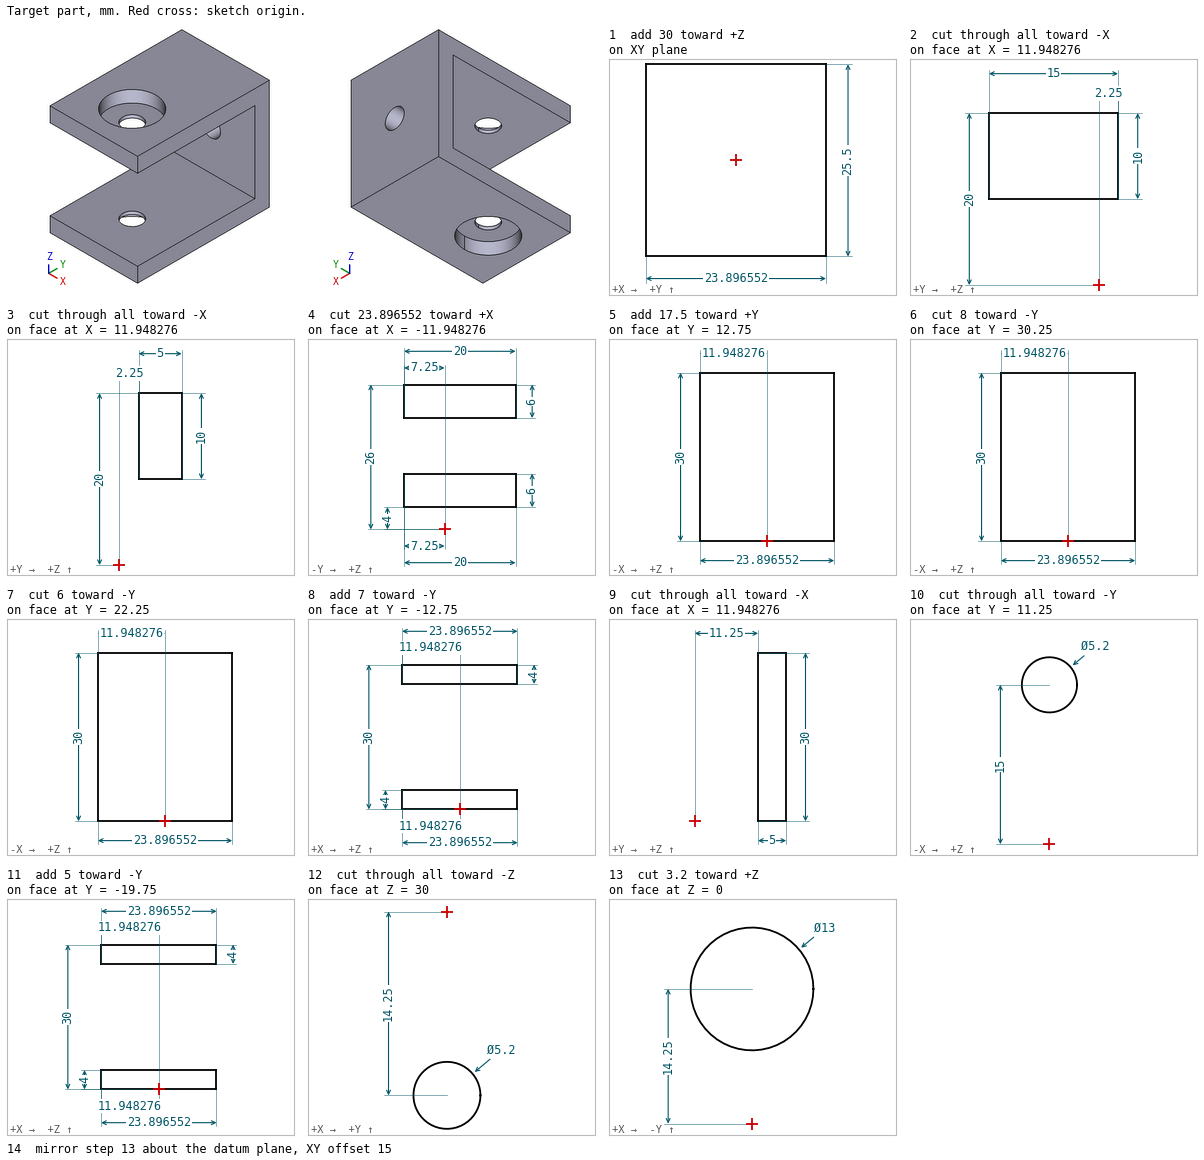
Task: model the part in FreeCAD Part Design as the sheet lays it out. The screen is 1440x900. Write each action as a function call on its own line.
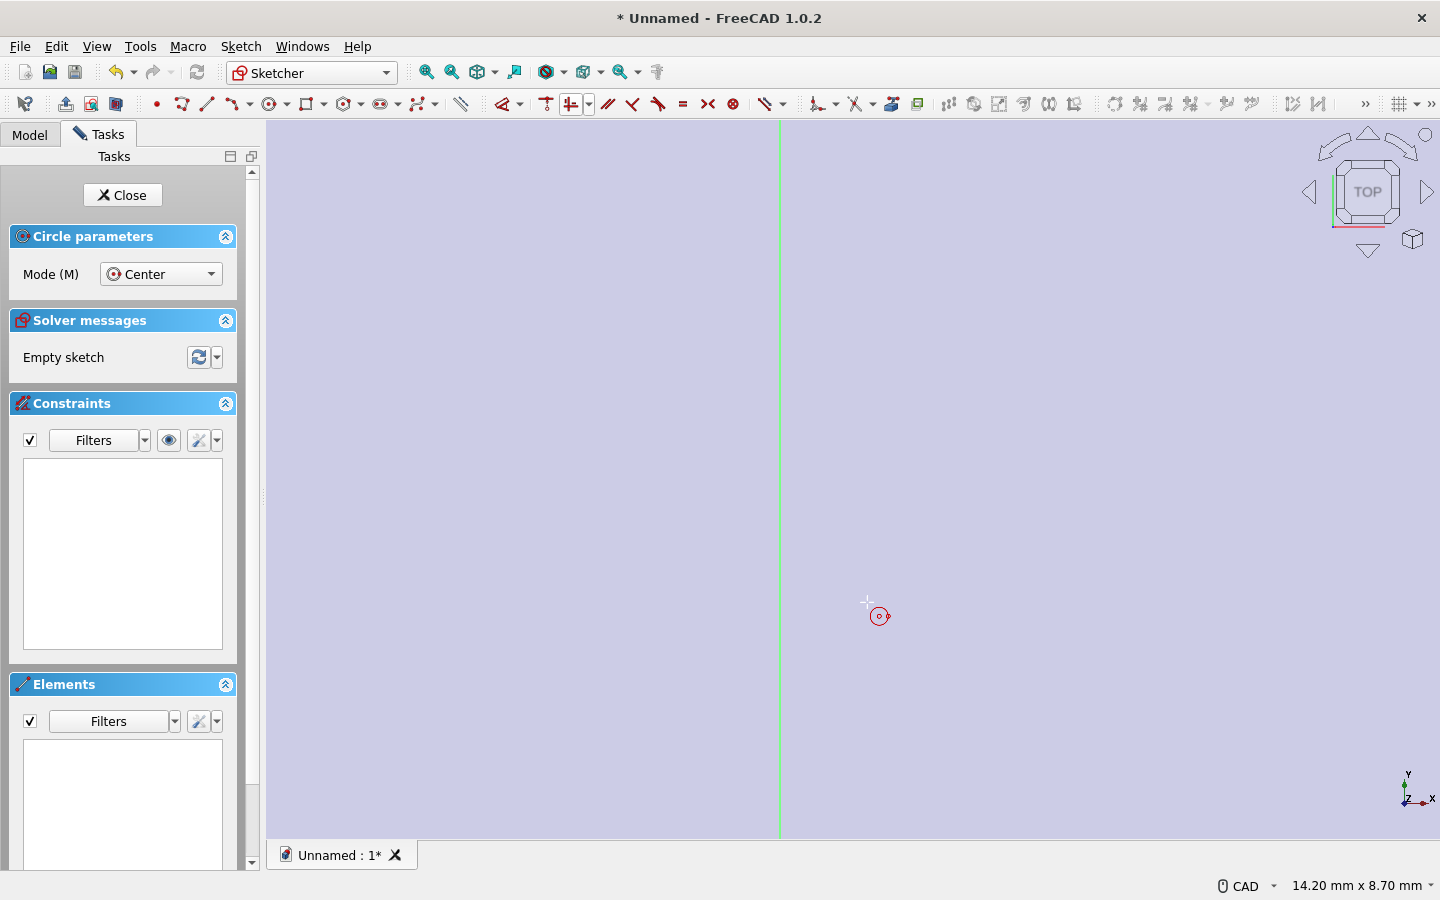
click(780, 478)
move(932, 326)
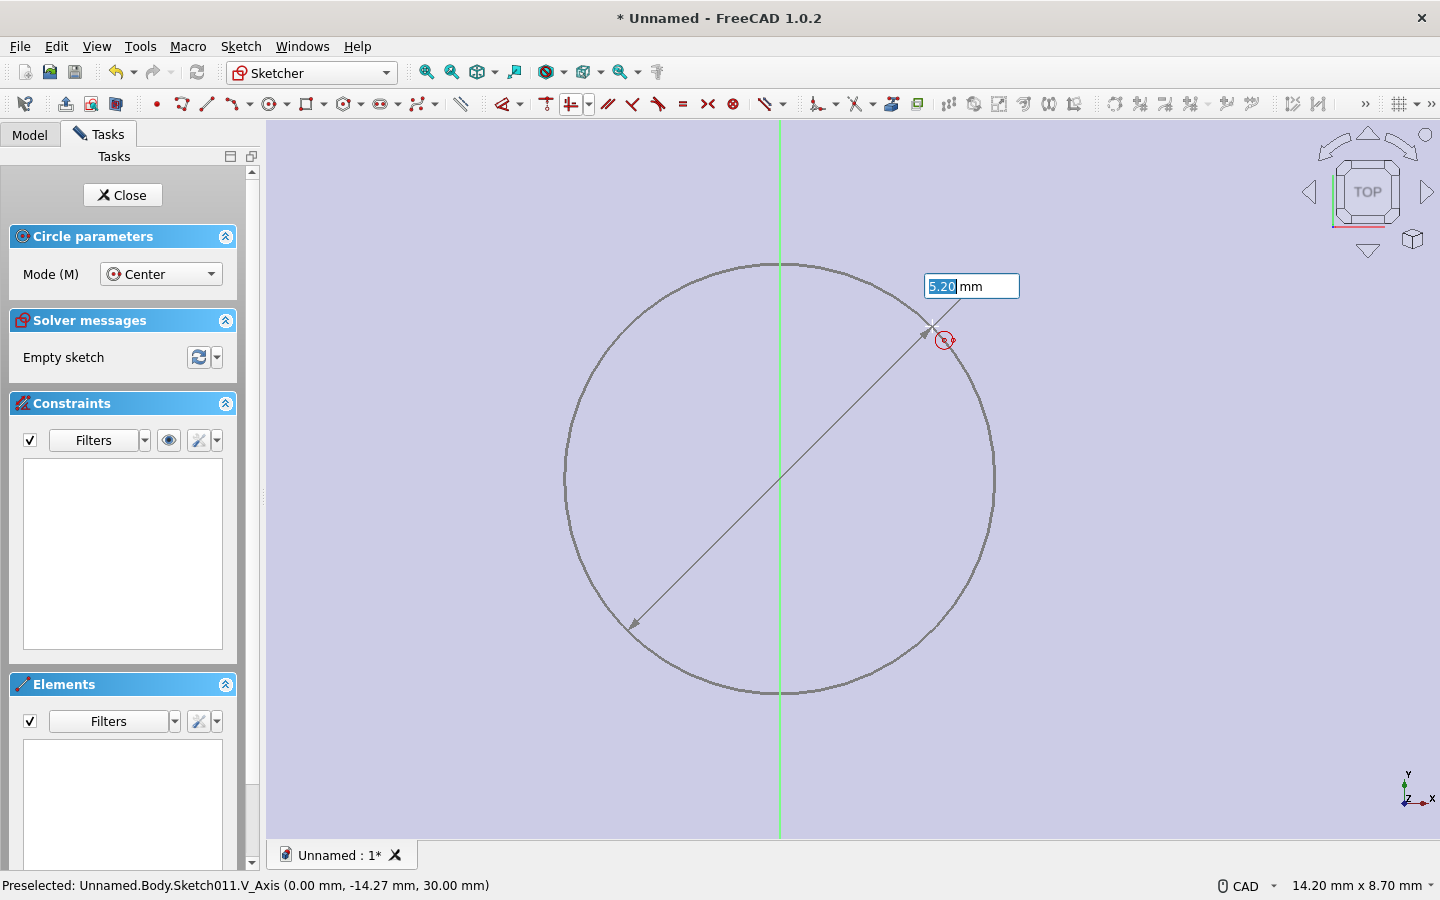
text(5.2)
key(Return)
key(Escape)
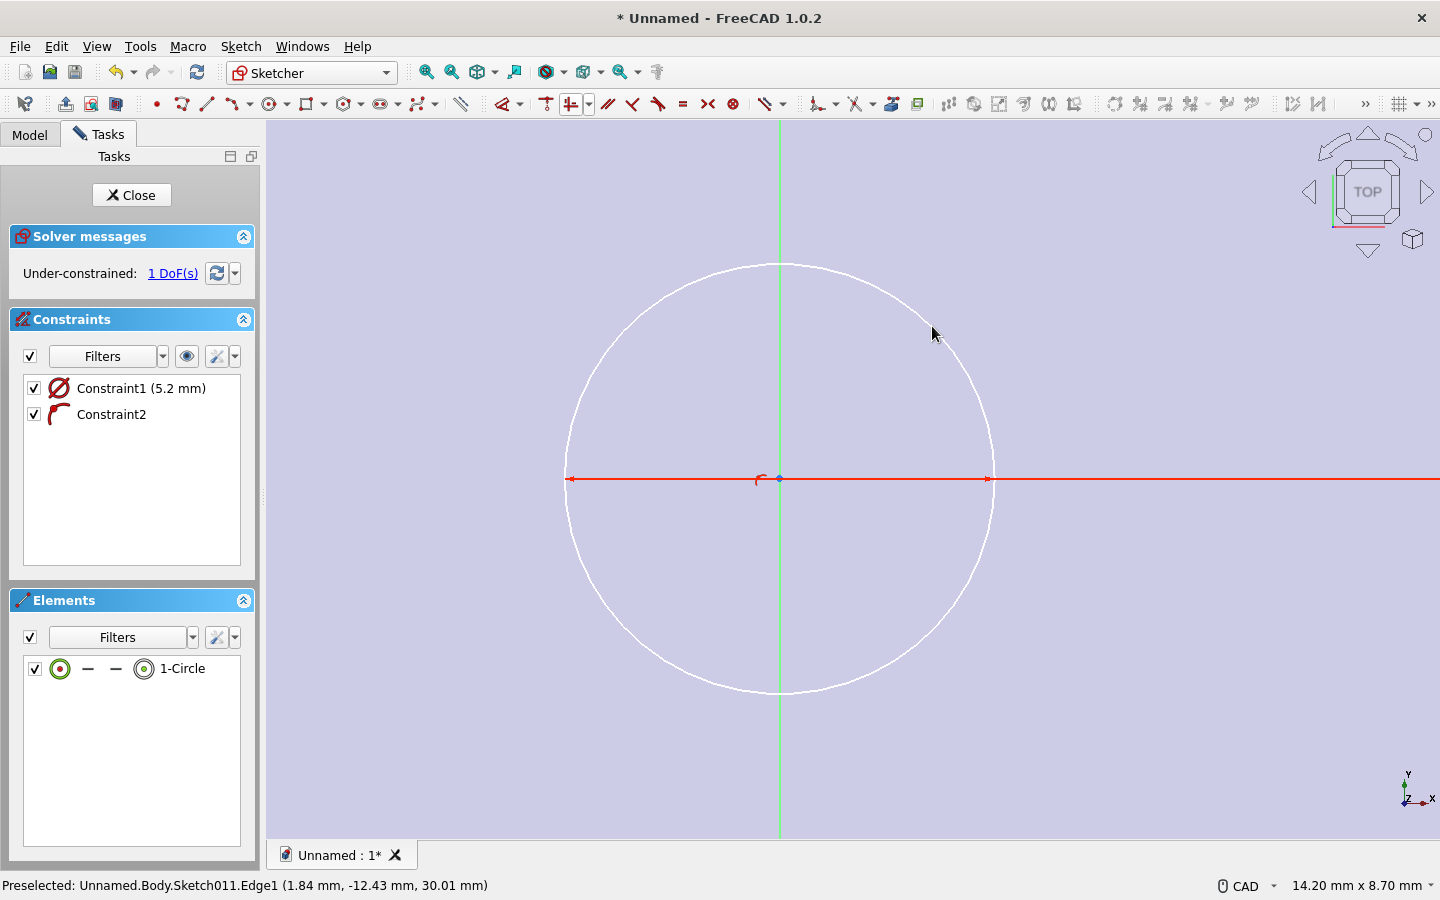
key(d)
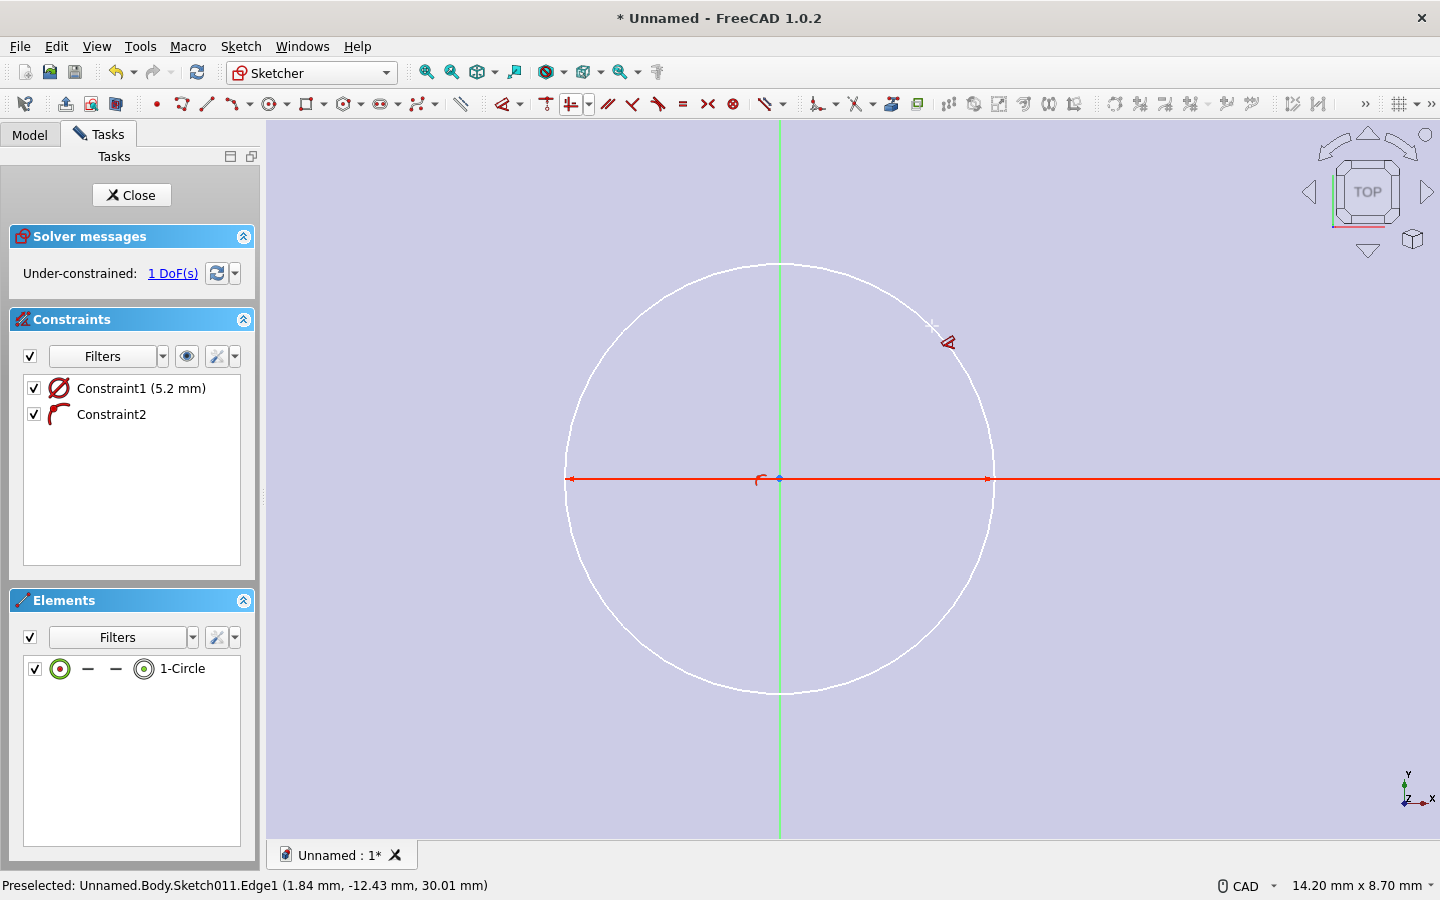
click(780, 479)
click(814, 314)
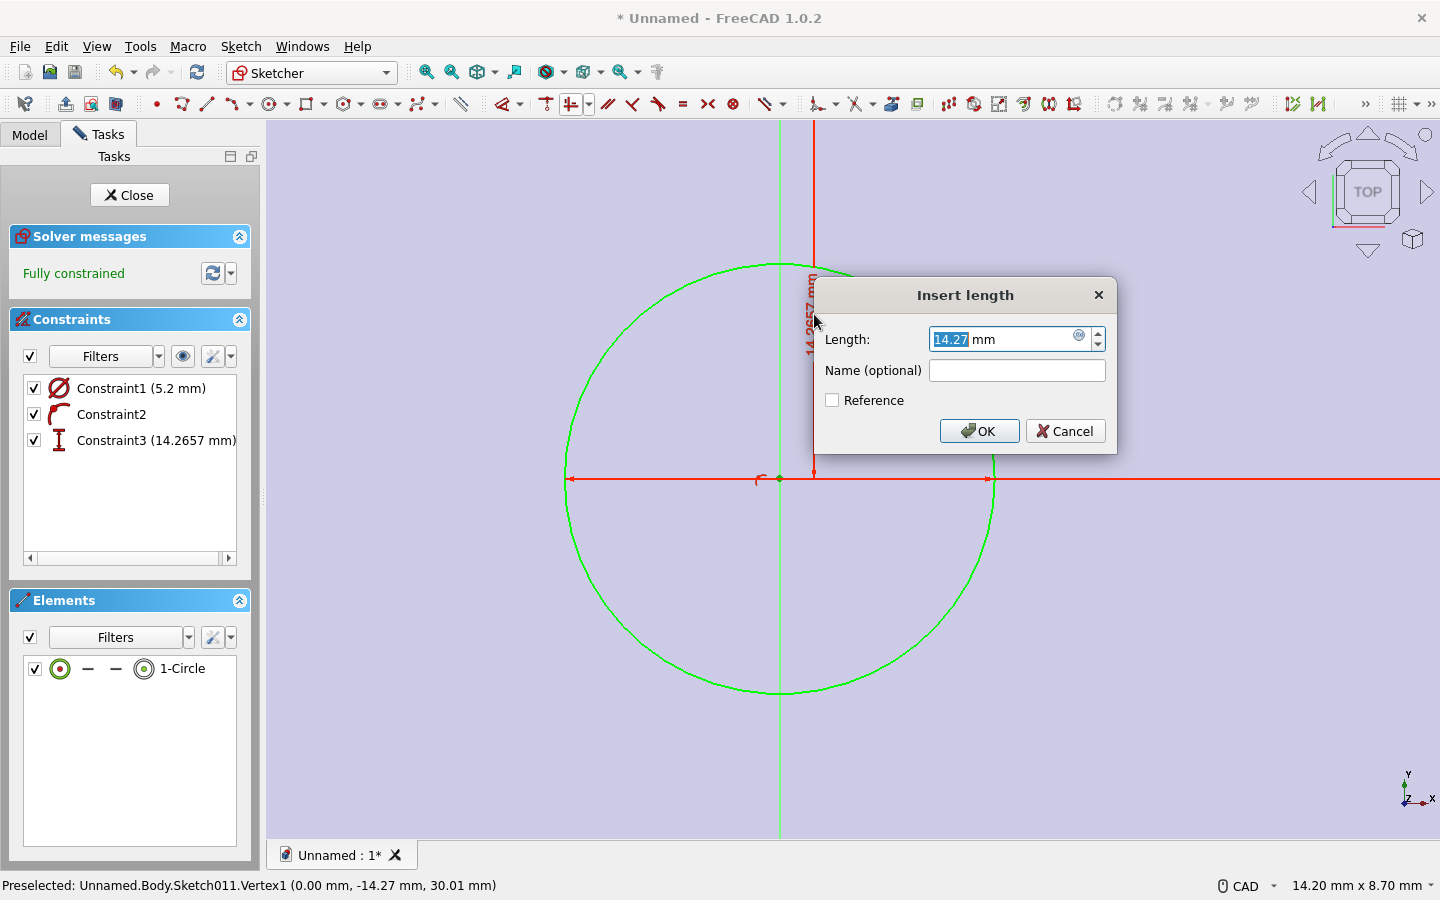
text(14.25)
key(Return)
key(Escape)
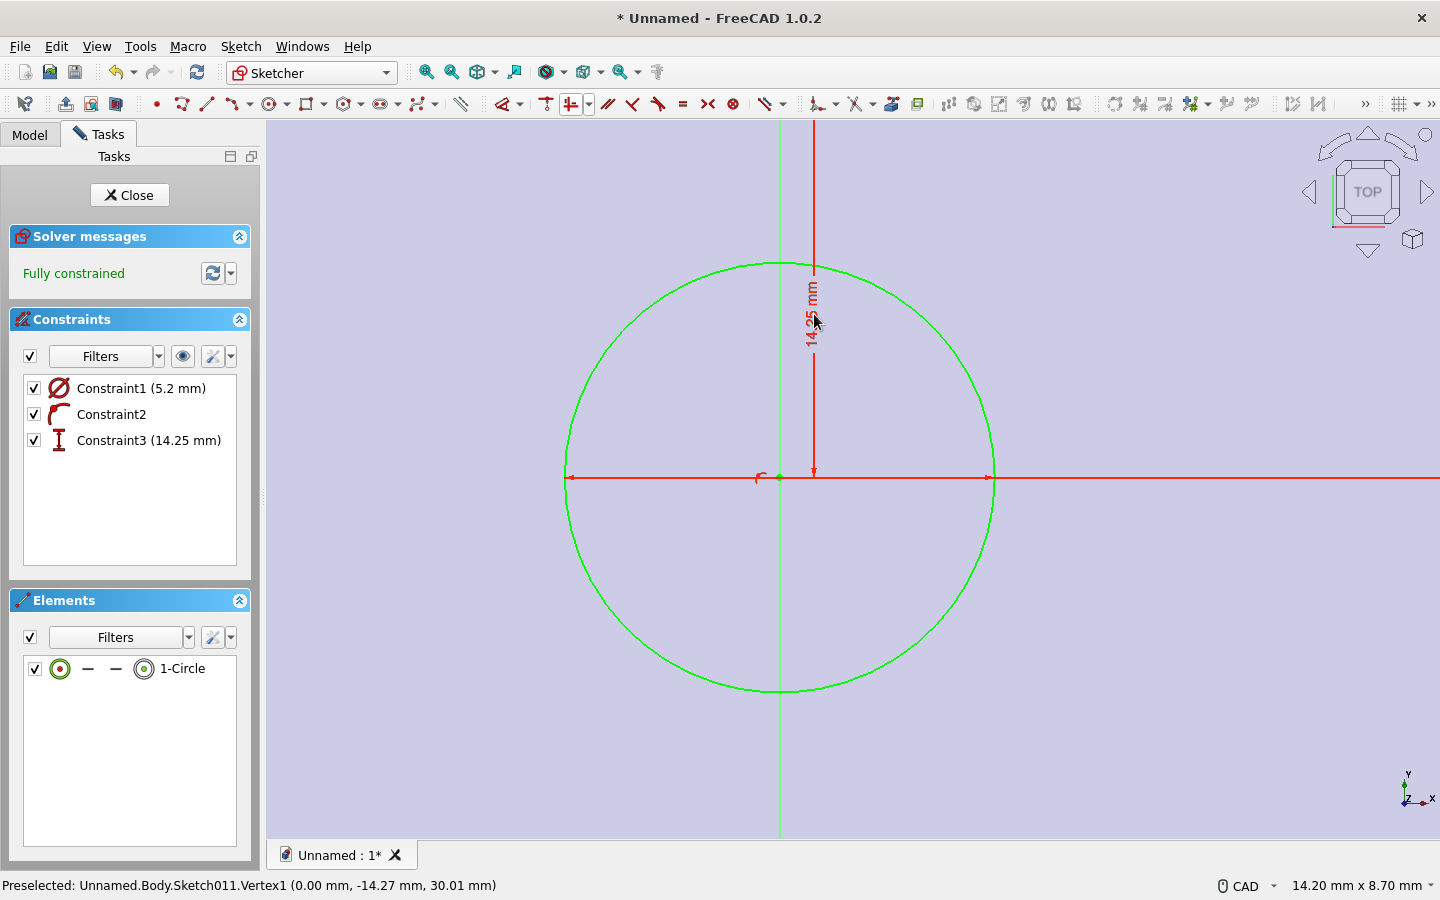
click(130, 195)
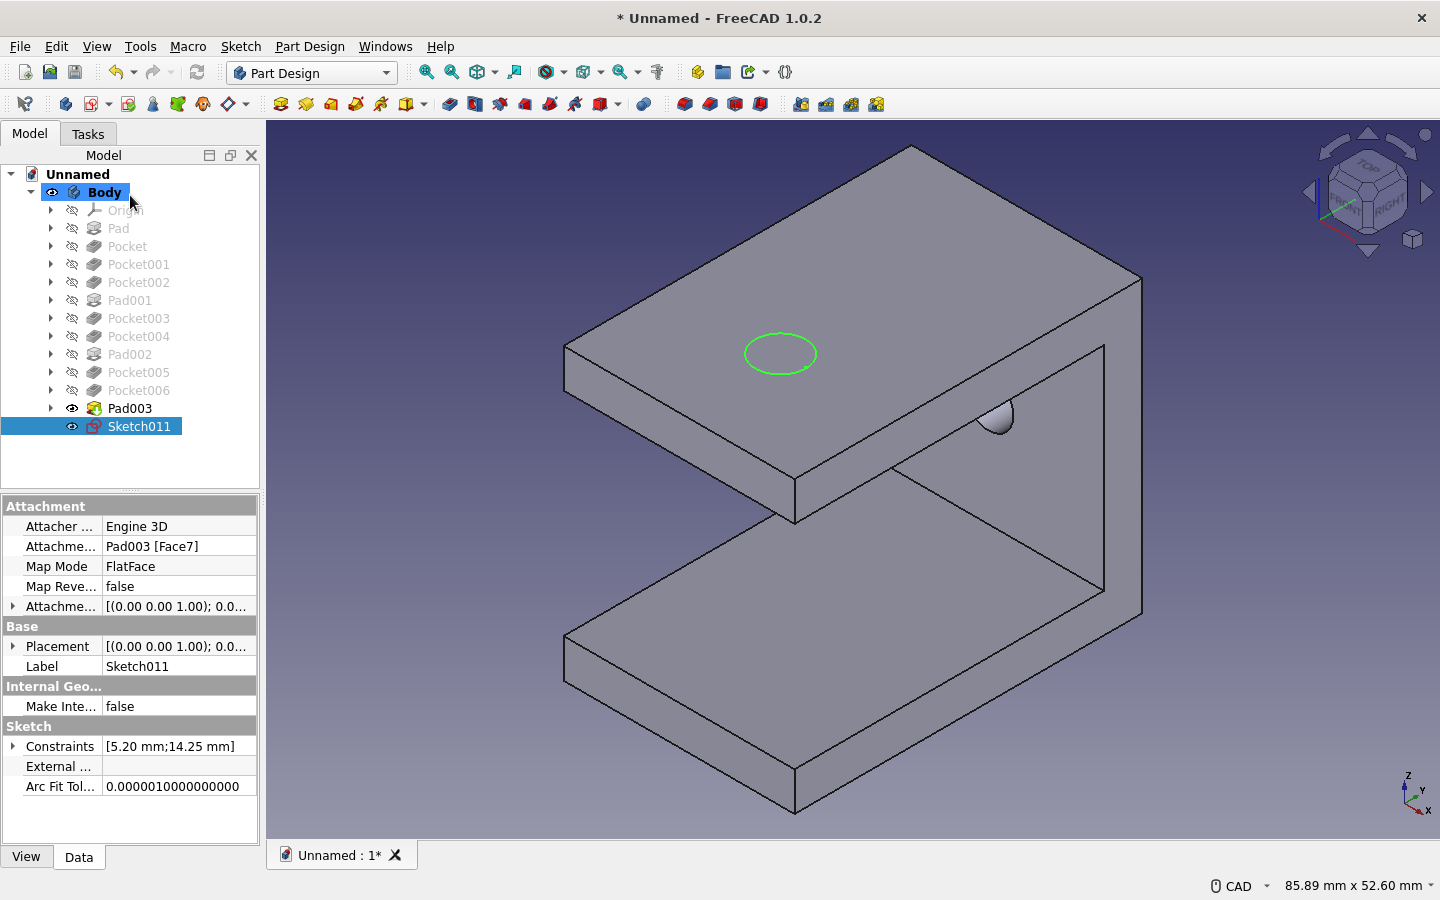
click(450, 104)